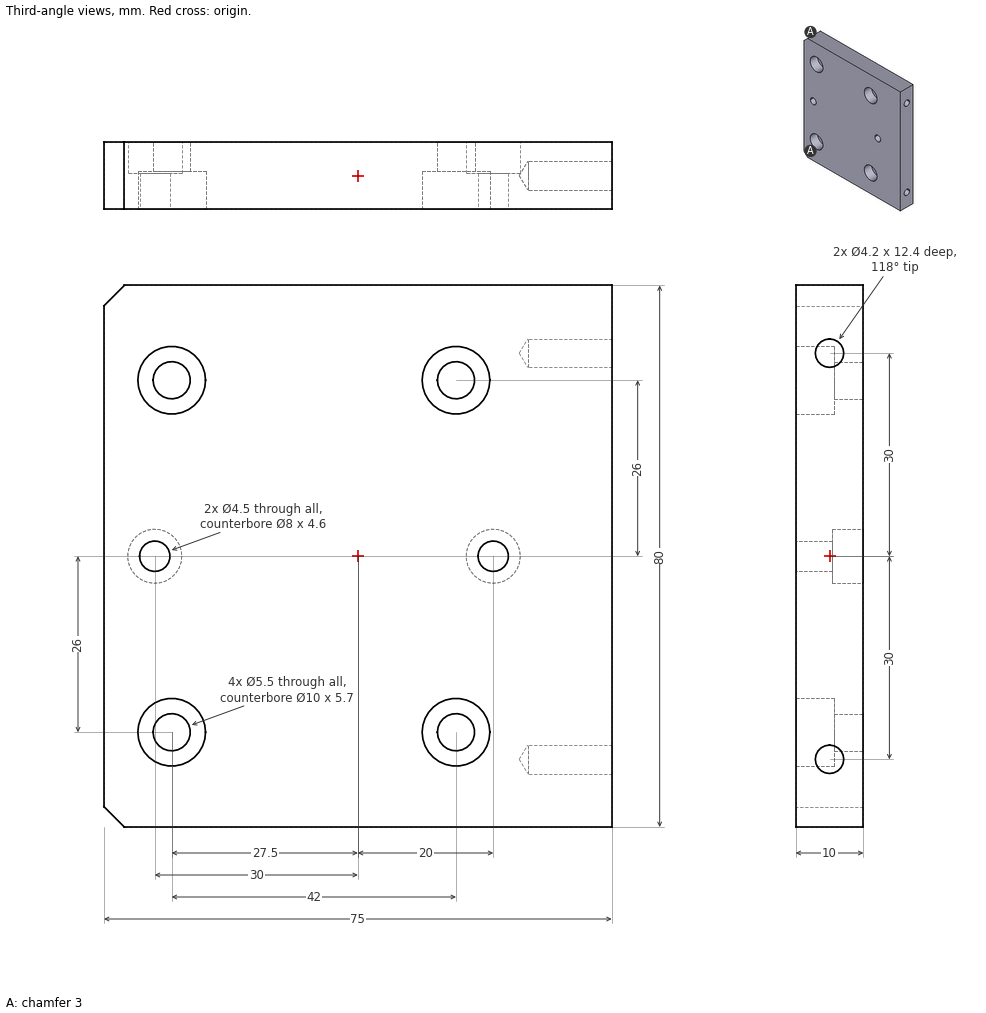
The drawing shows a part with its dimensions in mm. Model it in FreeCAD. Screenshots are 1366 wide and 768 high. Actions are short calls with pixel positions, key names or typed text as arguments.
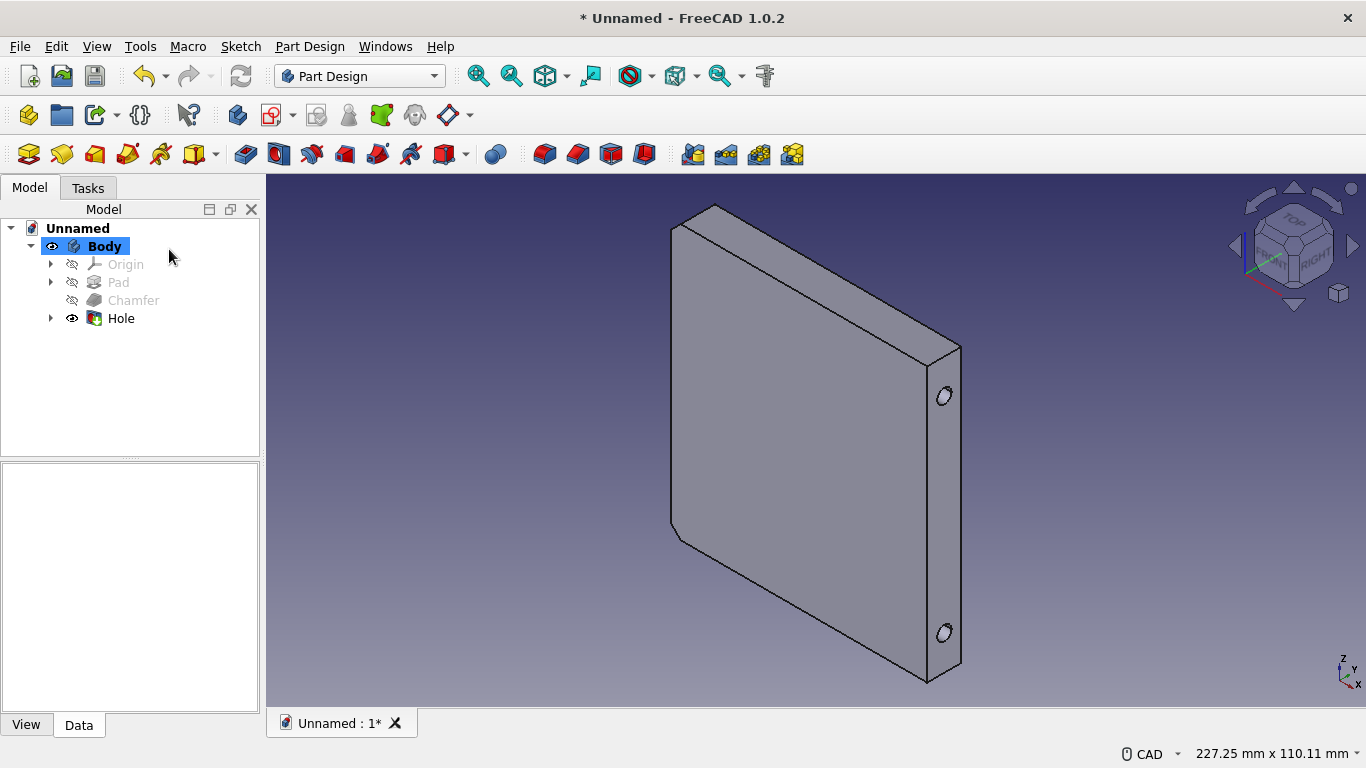
click(799, 449)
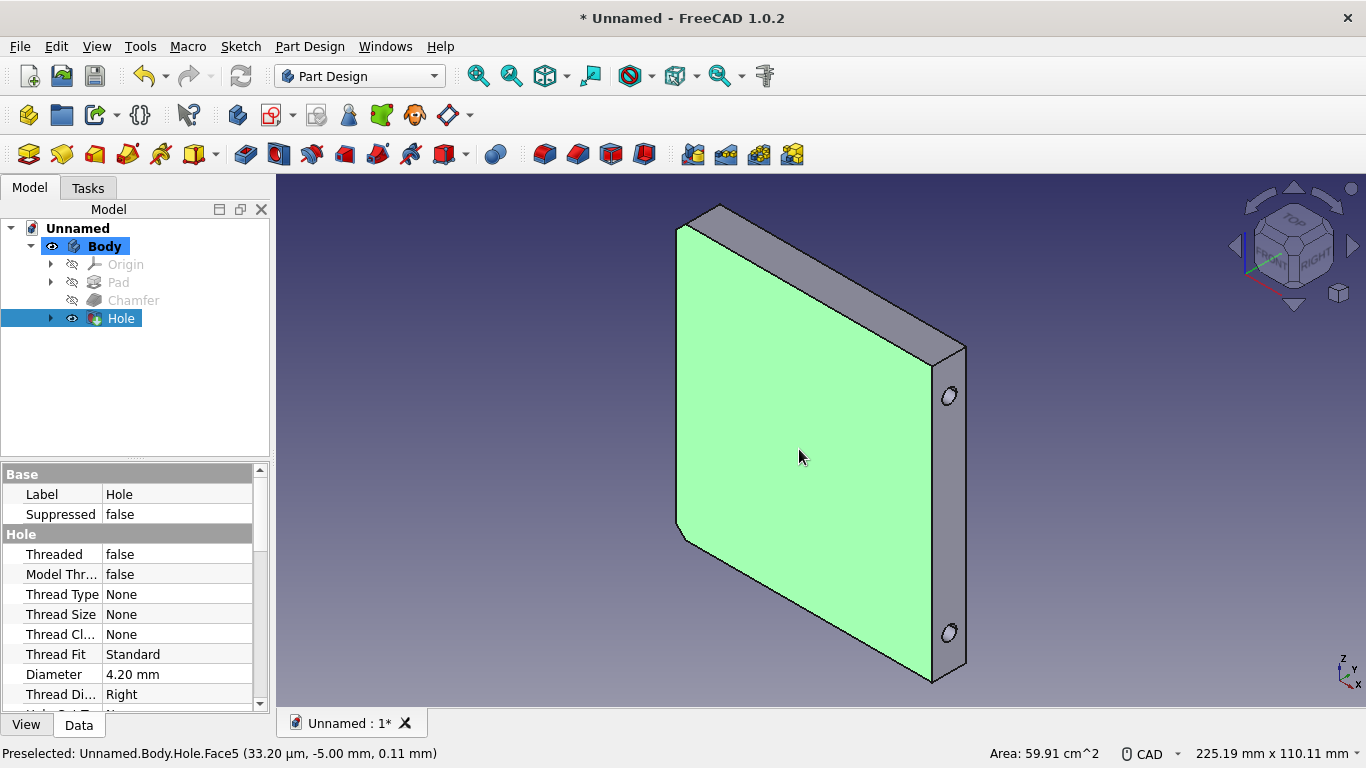
click(270, 116)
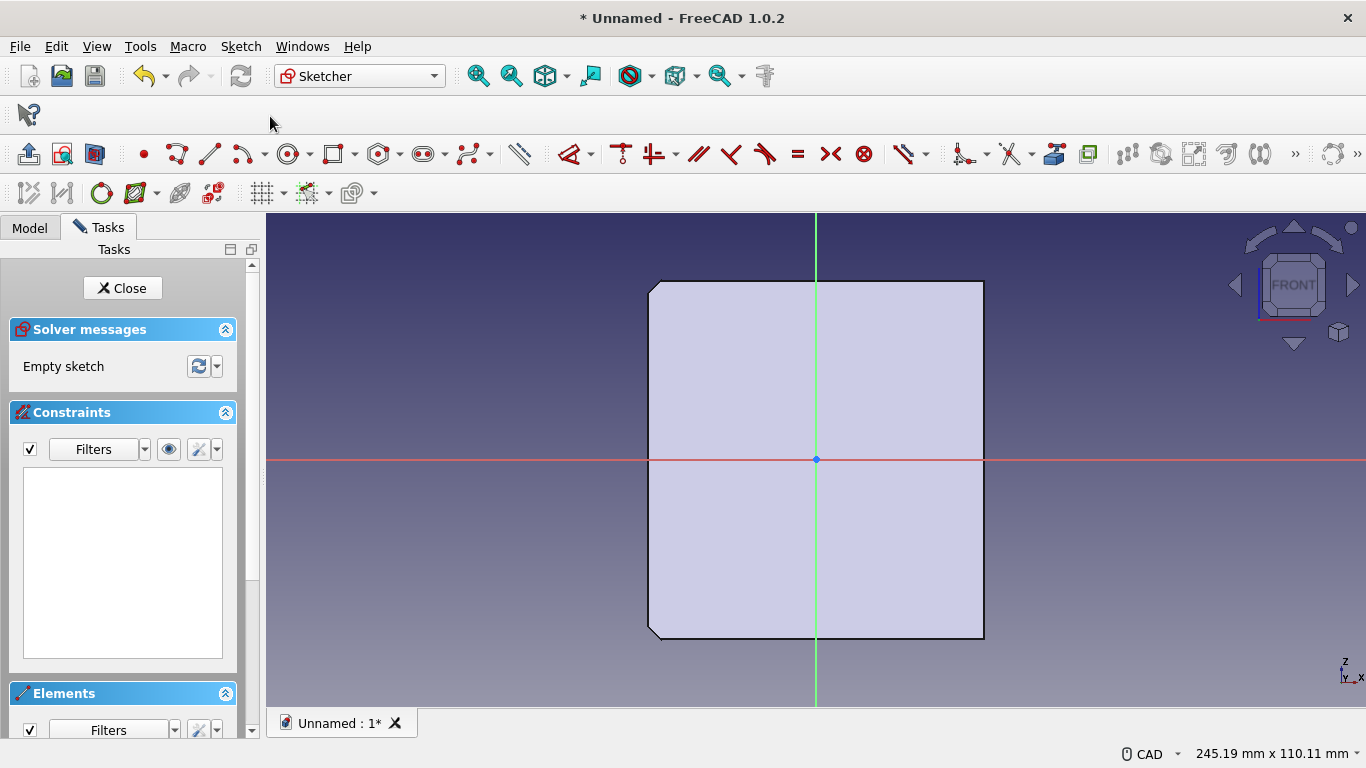
click(288, 154)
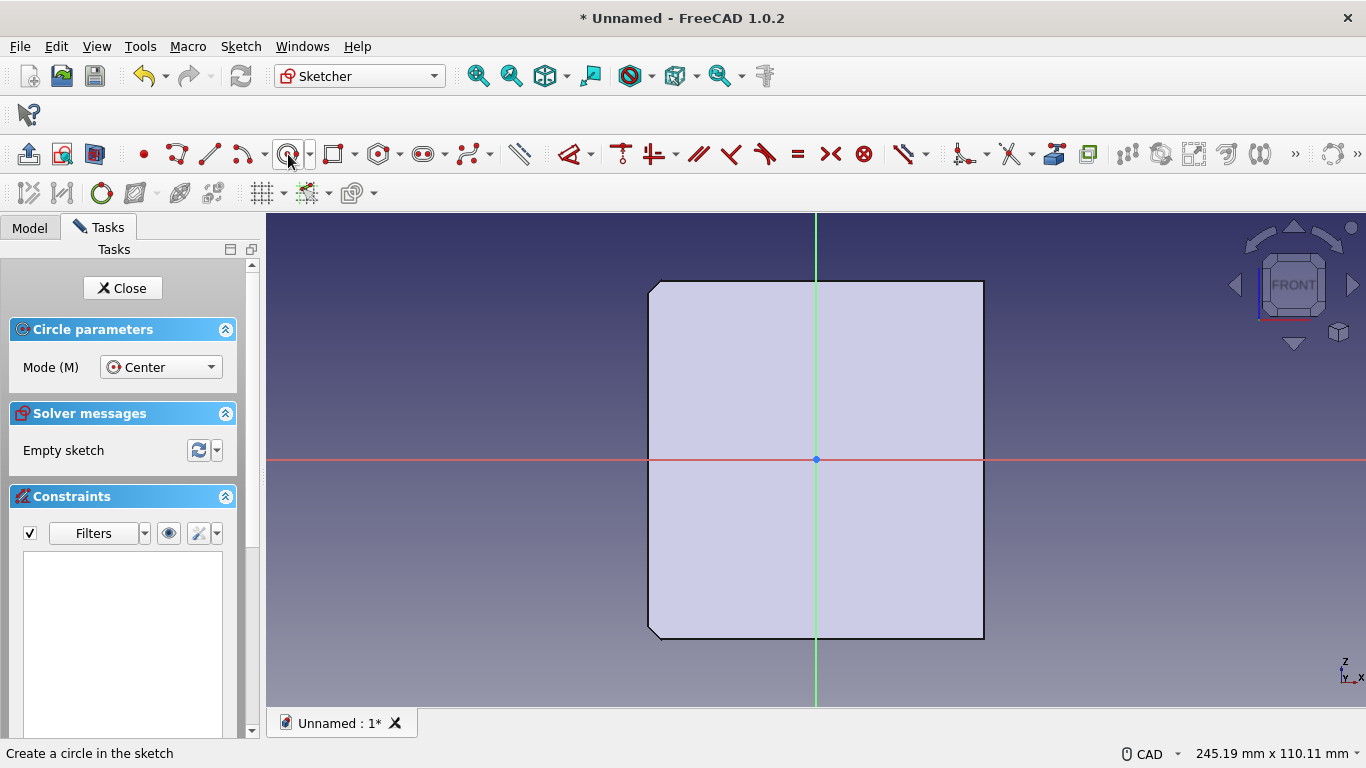
scroll(693, 577, up, 4)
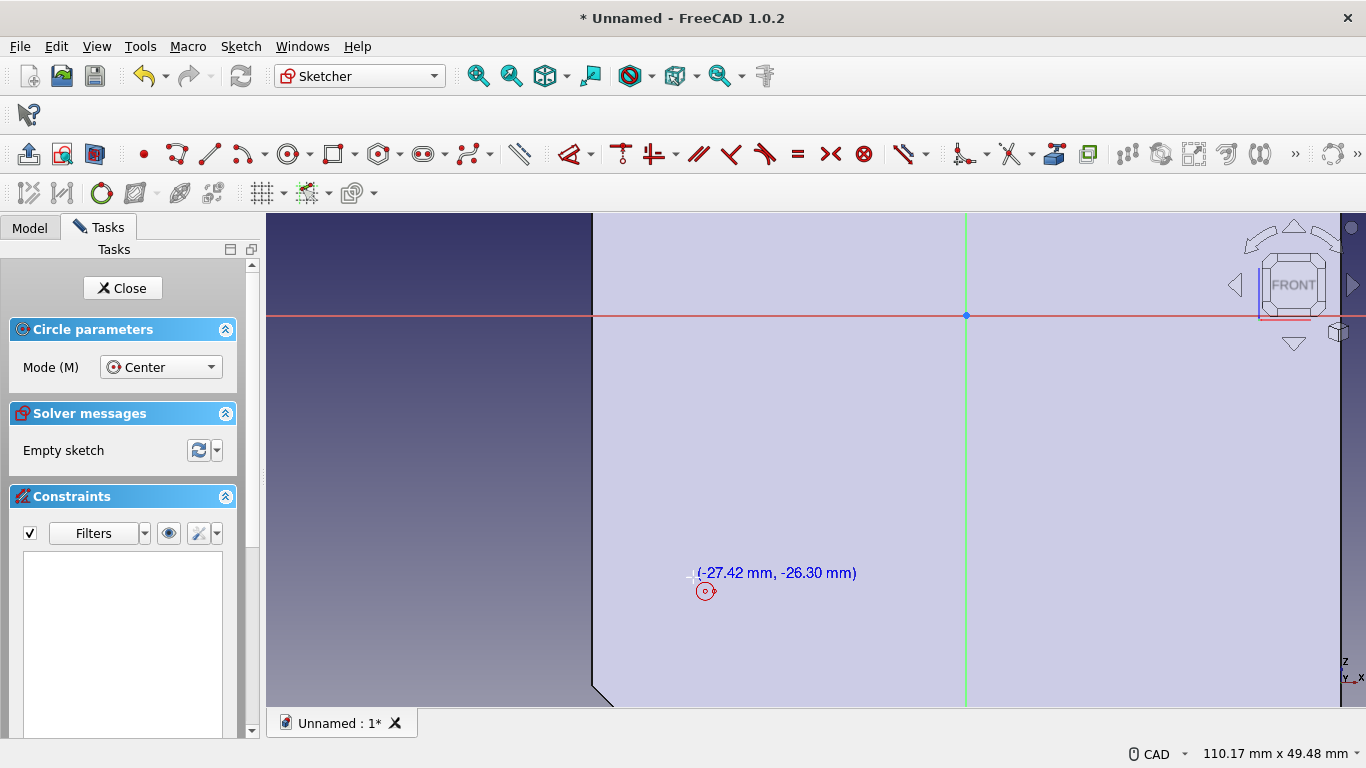
click(692, 575)
click(711, 556)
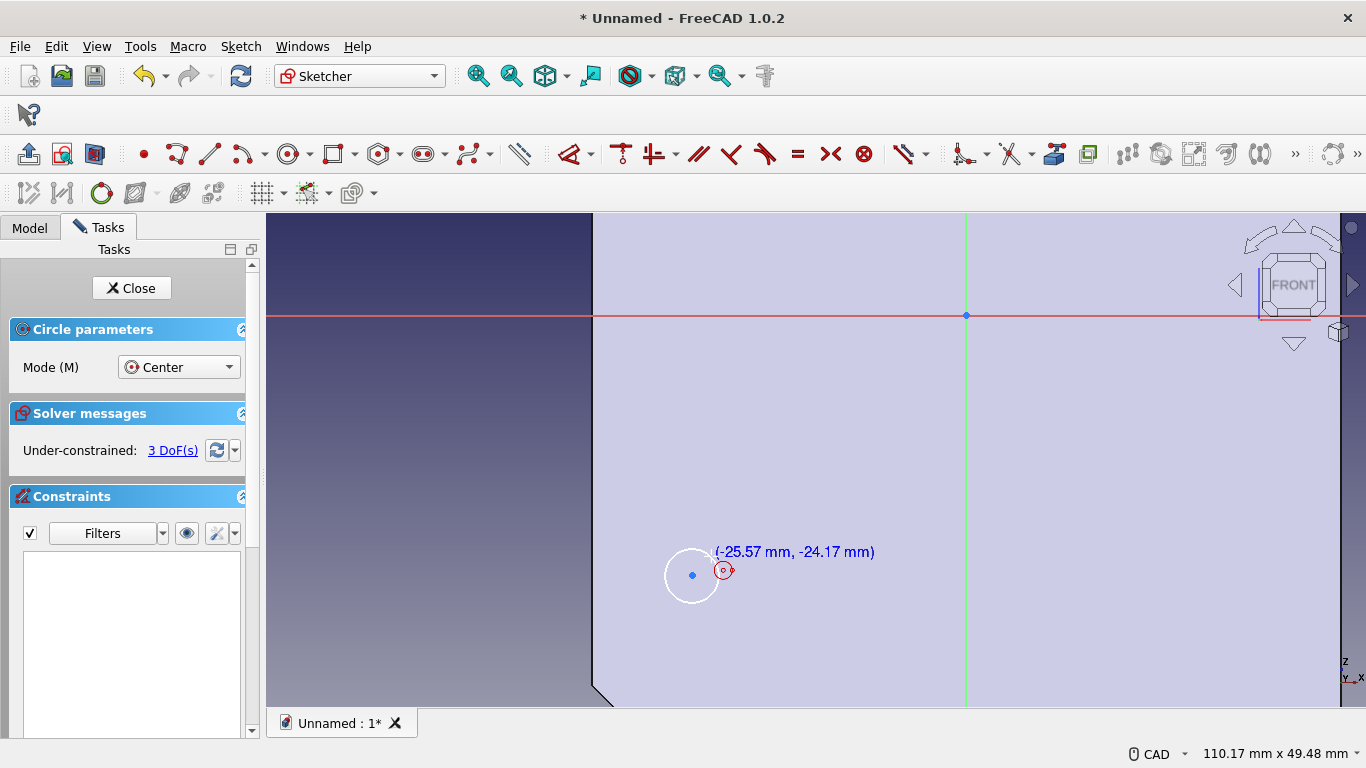
click(1111, 575)
click(1130, 556)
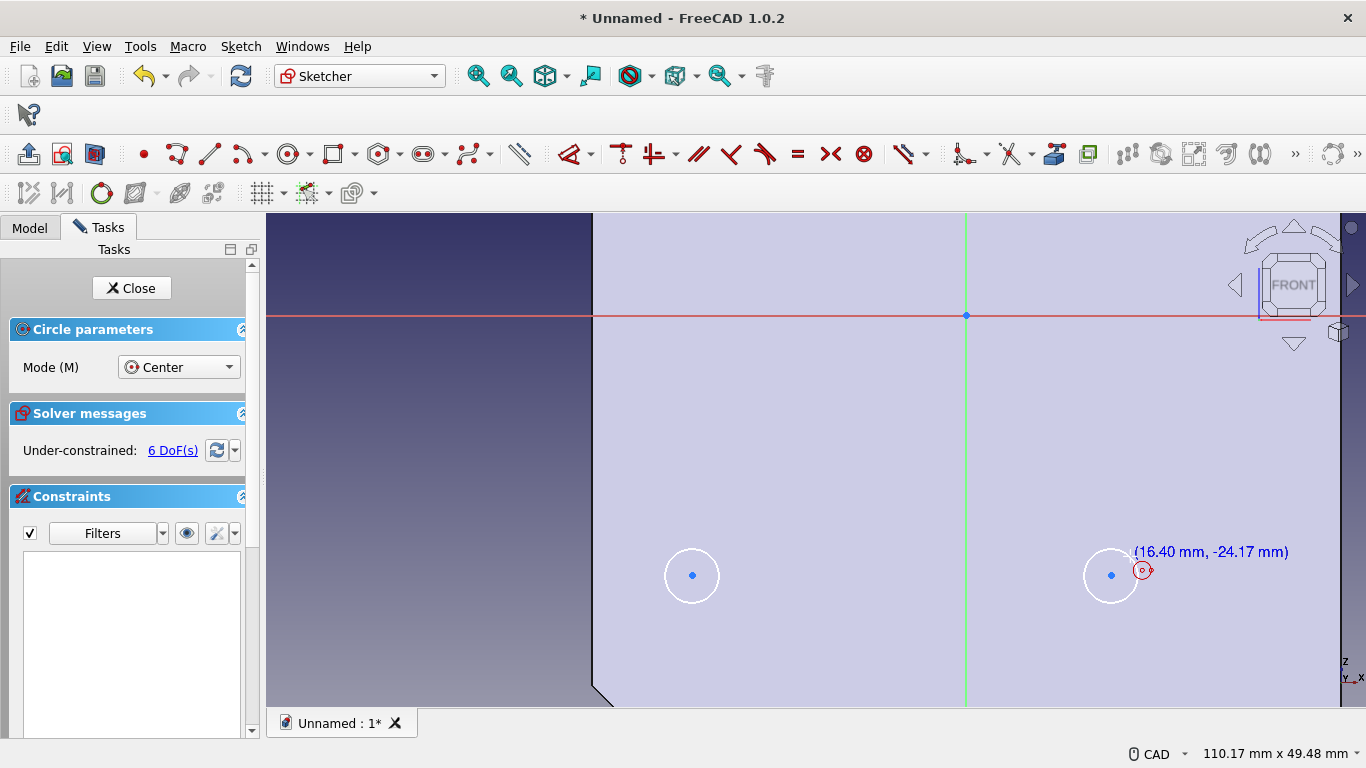
scroll(560, 636, down, 3)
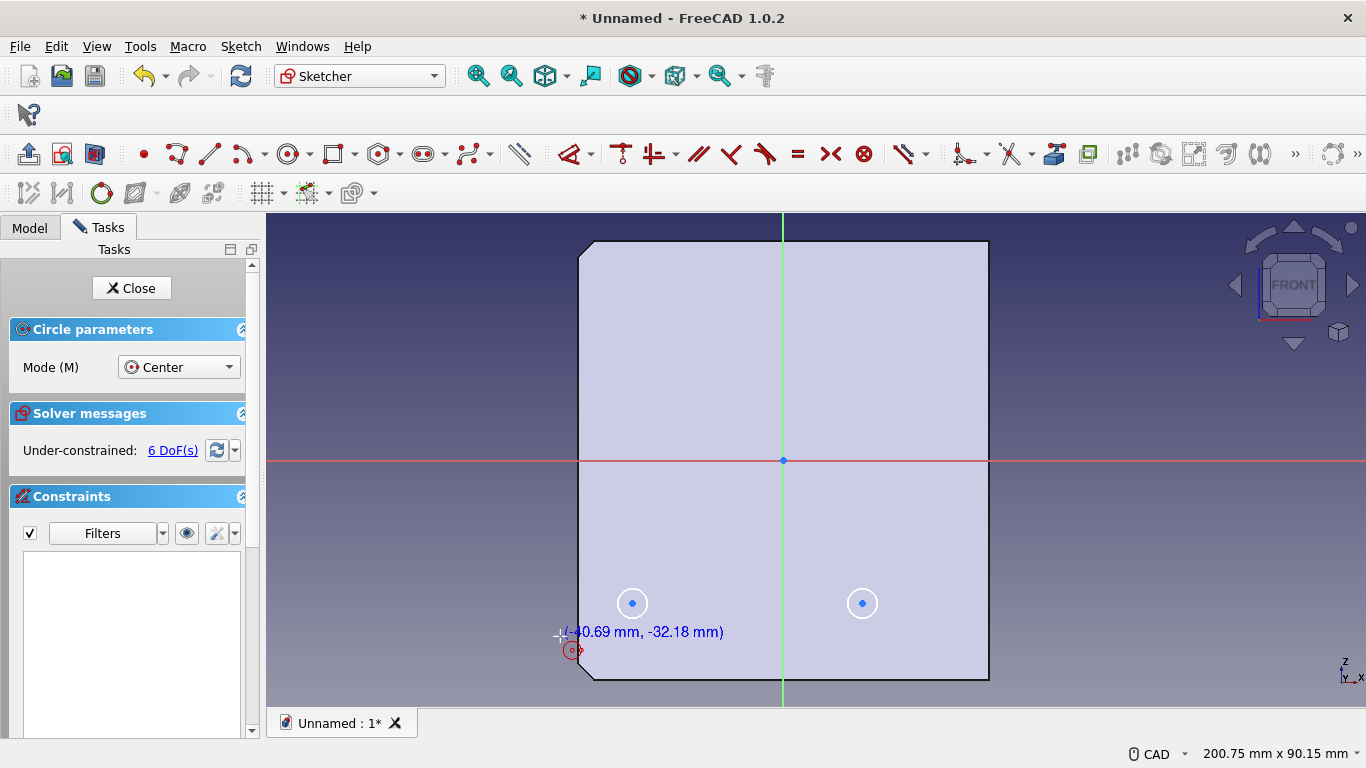
scroll(863, 318, up, 3)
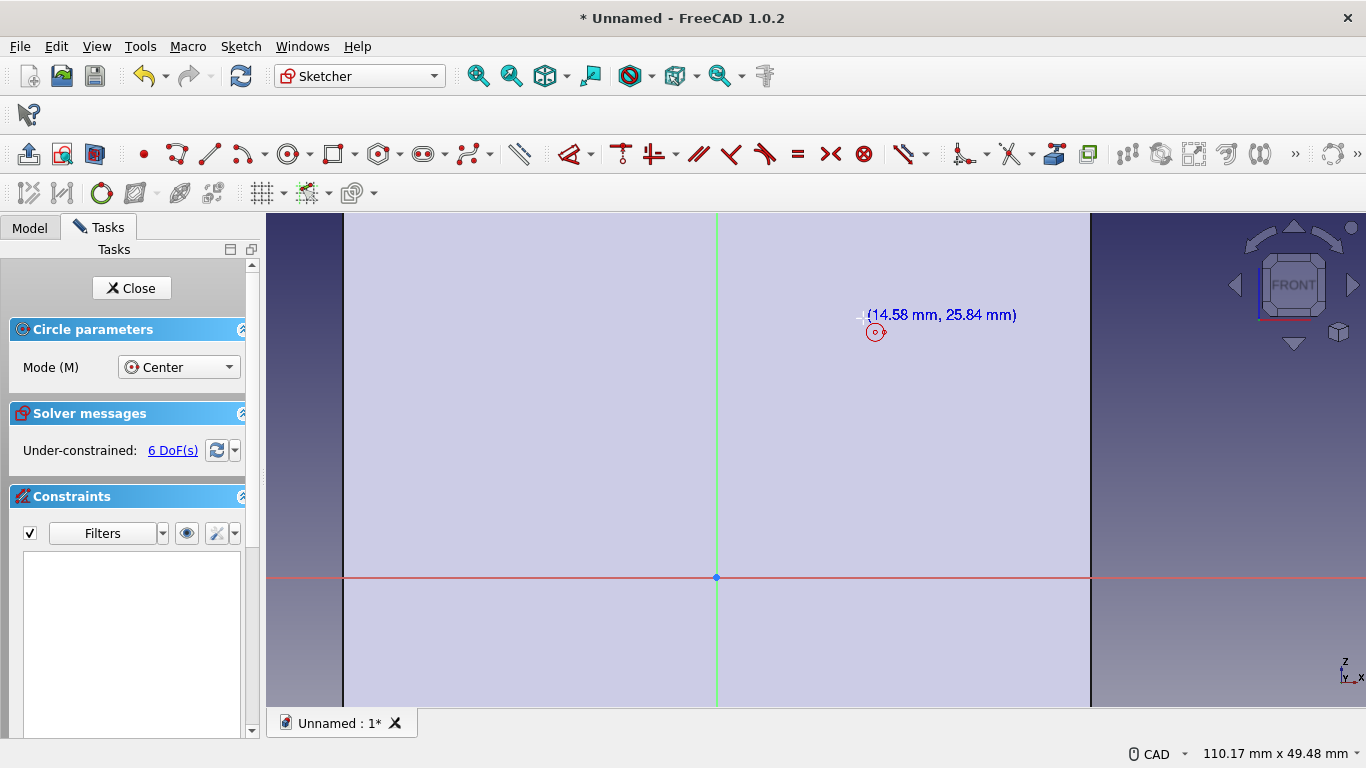
click(862, 318)
click(881, 299)